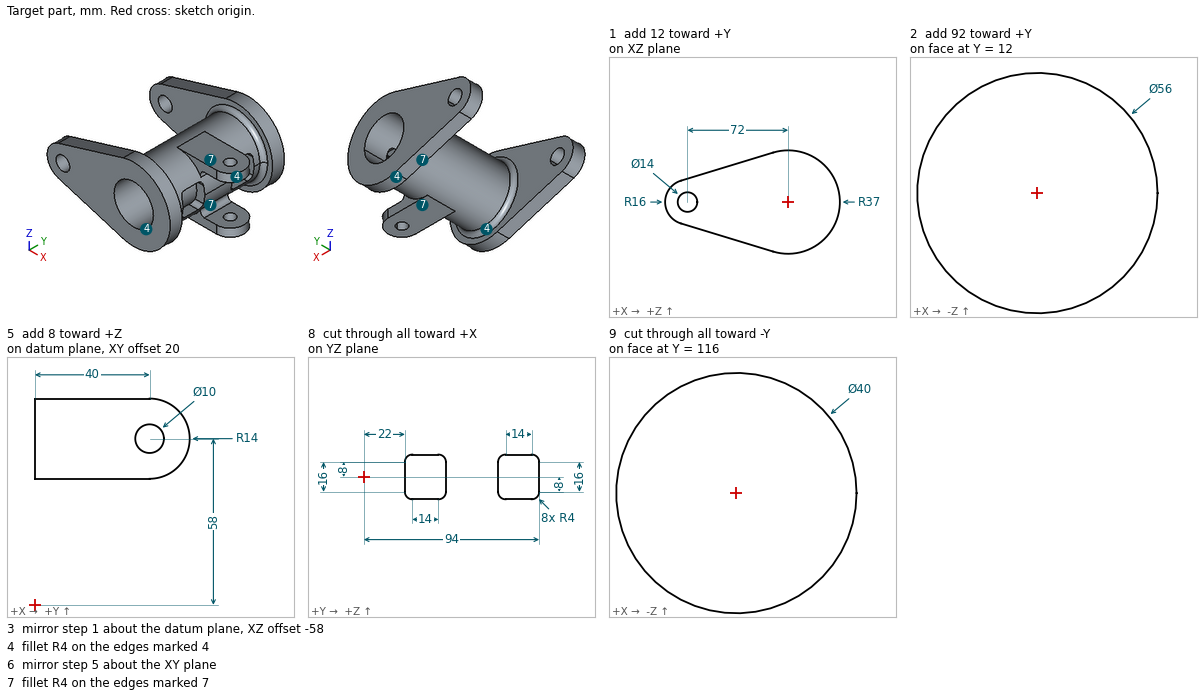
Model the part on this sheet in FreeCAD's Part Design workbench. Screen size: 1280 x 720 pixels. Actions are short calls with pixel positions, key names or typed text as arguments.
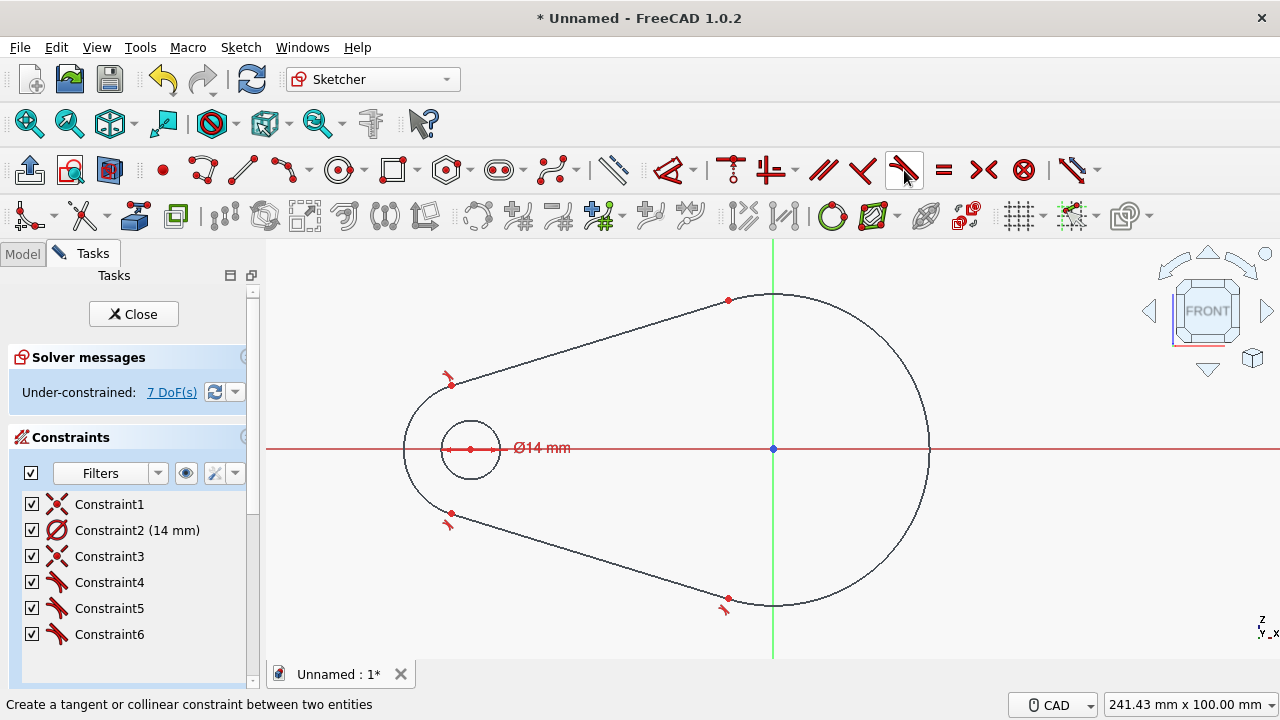
click(534, 361)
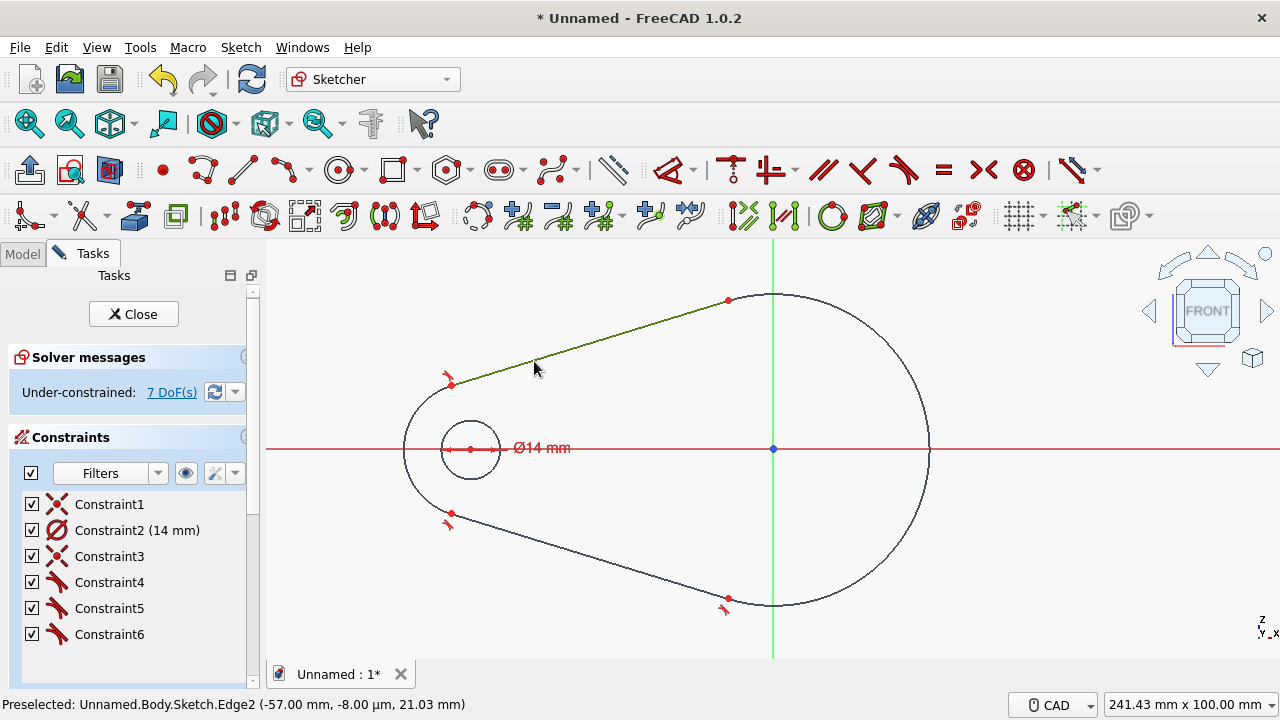
click(888, 556)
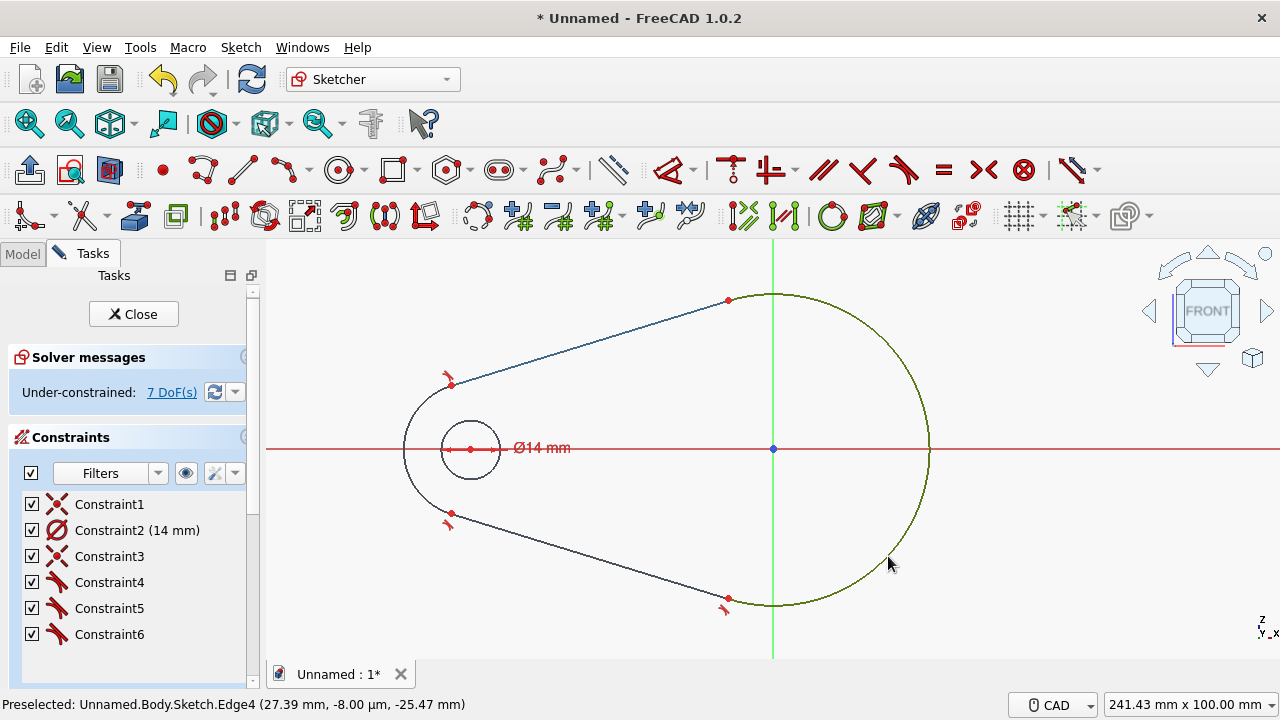
click(904, 170)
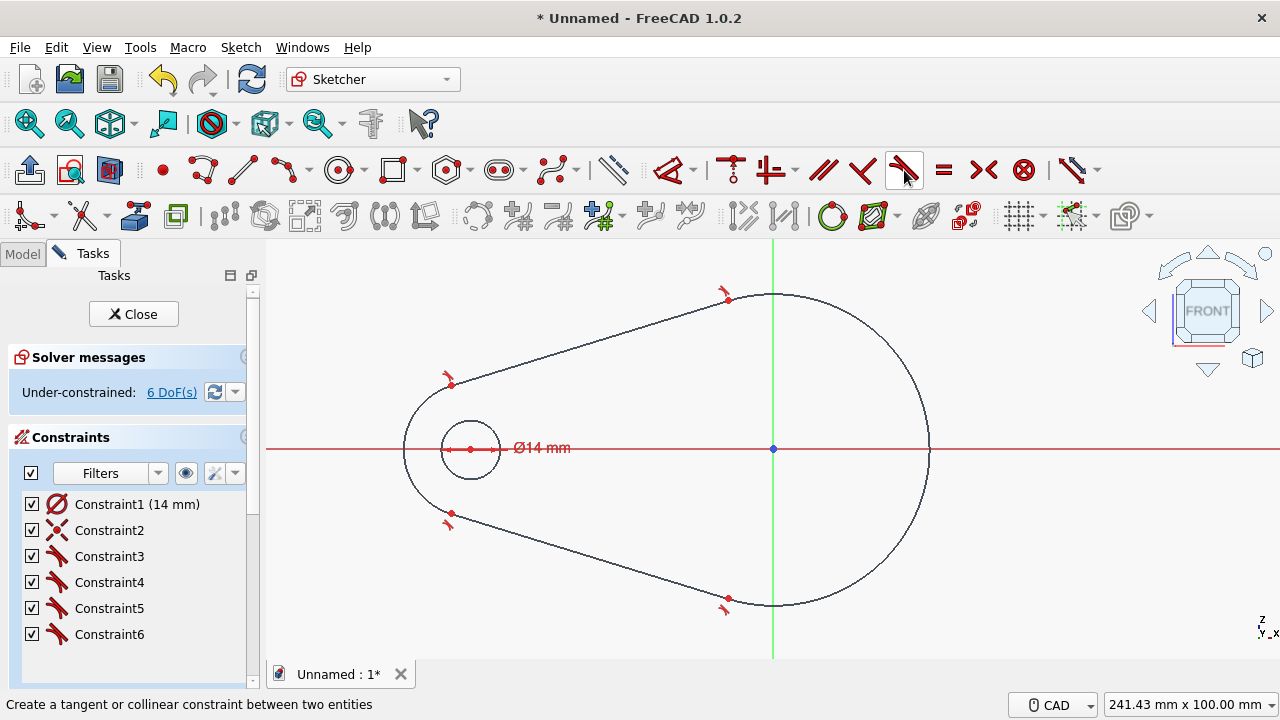
scroll(773, 449, up, 2)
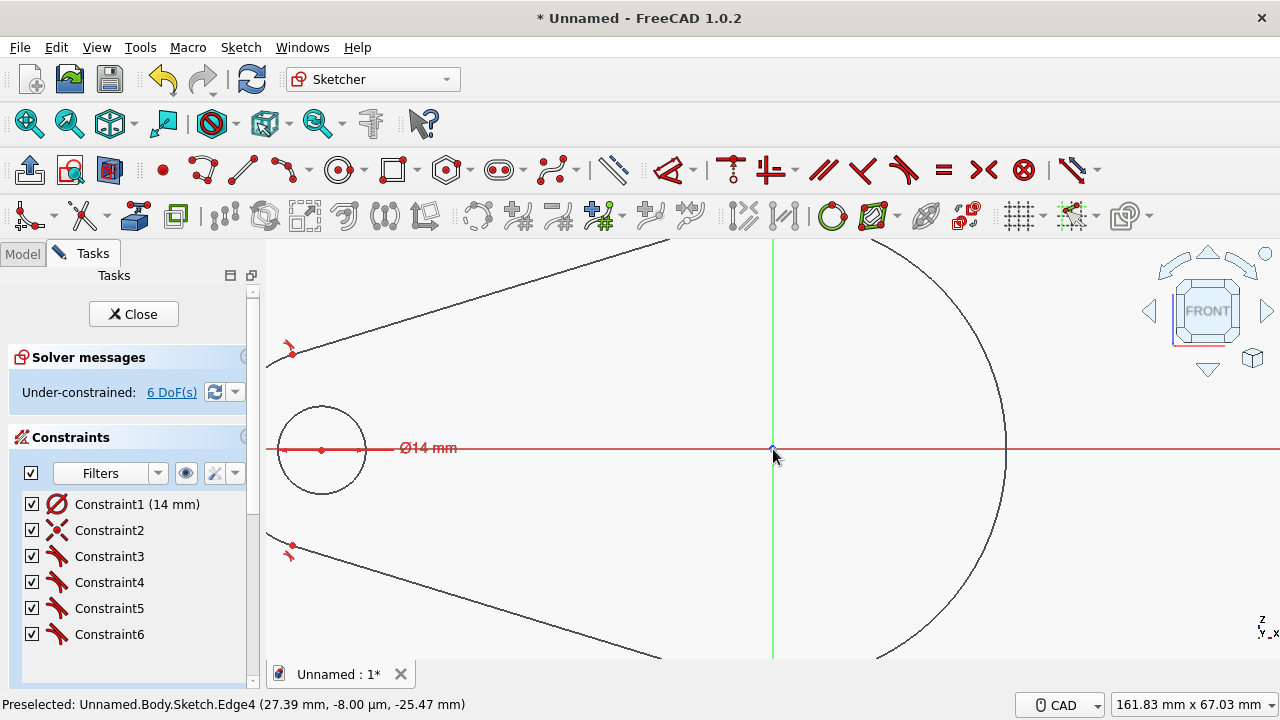
drag(763, 439, 784, 460)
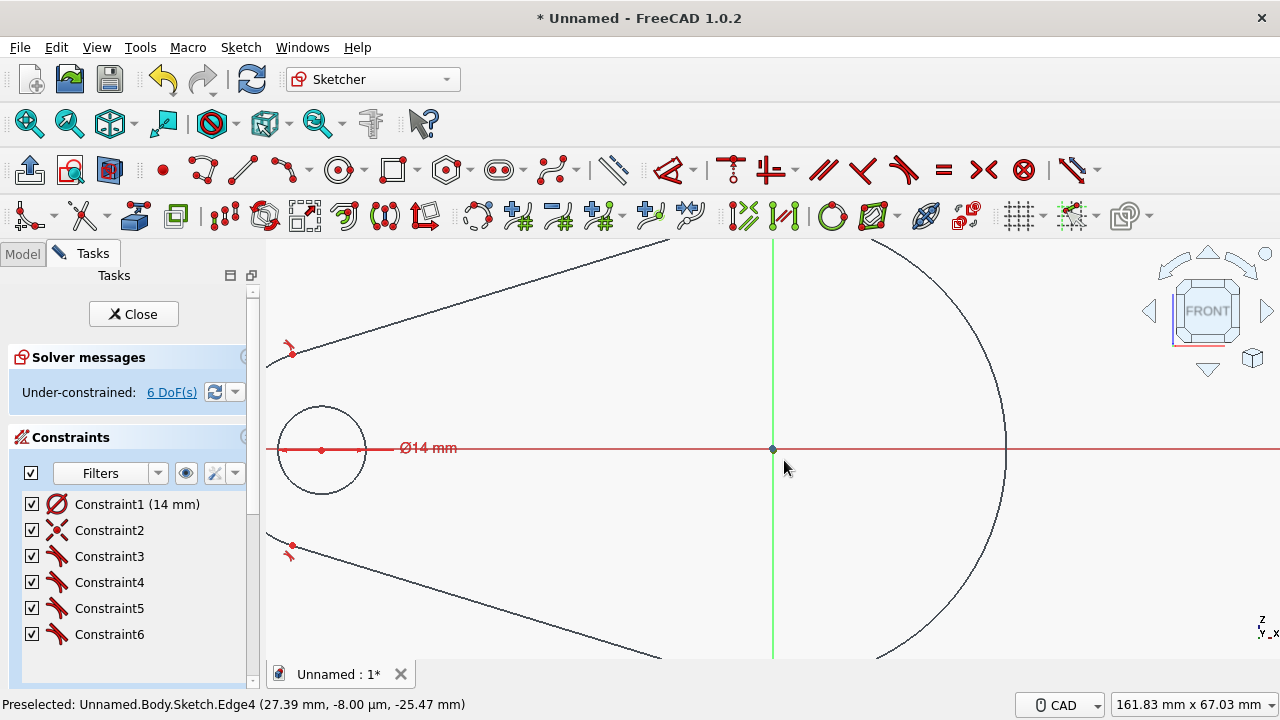
click(732, 170)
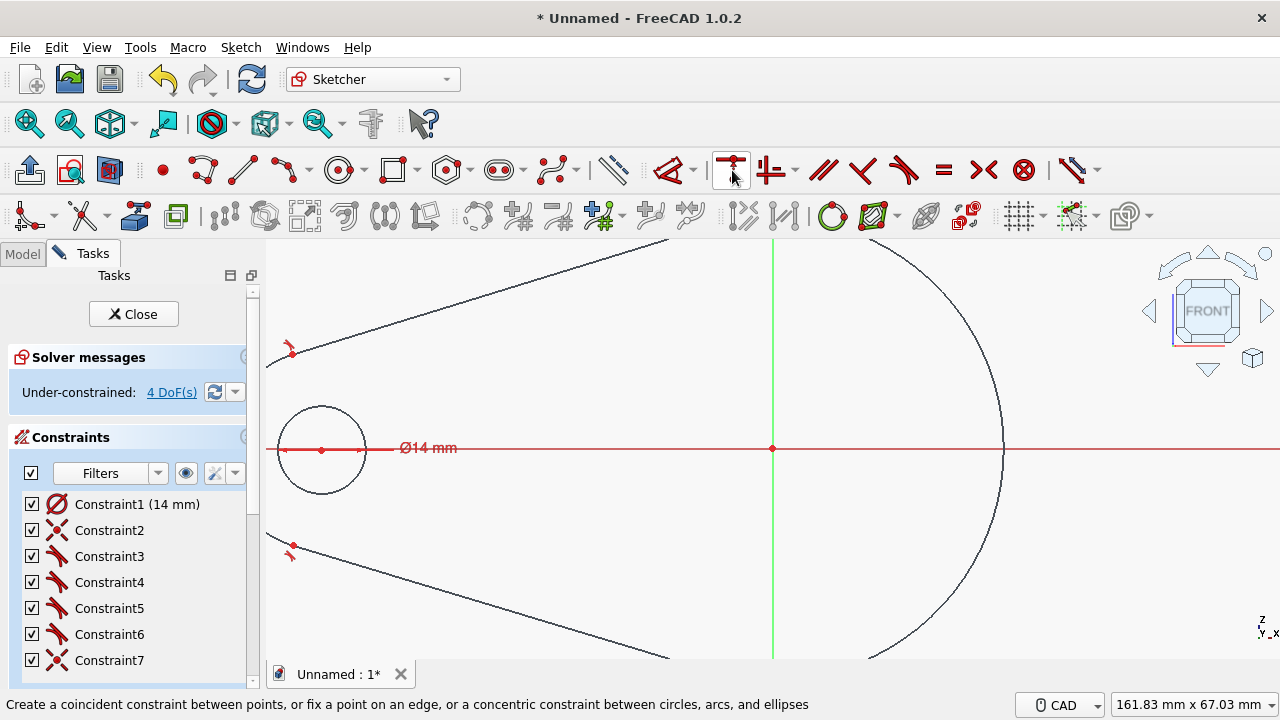
click(322, 450)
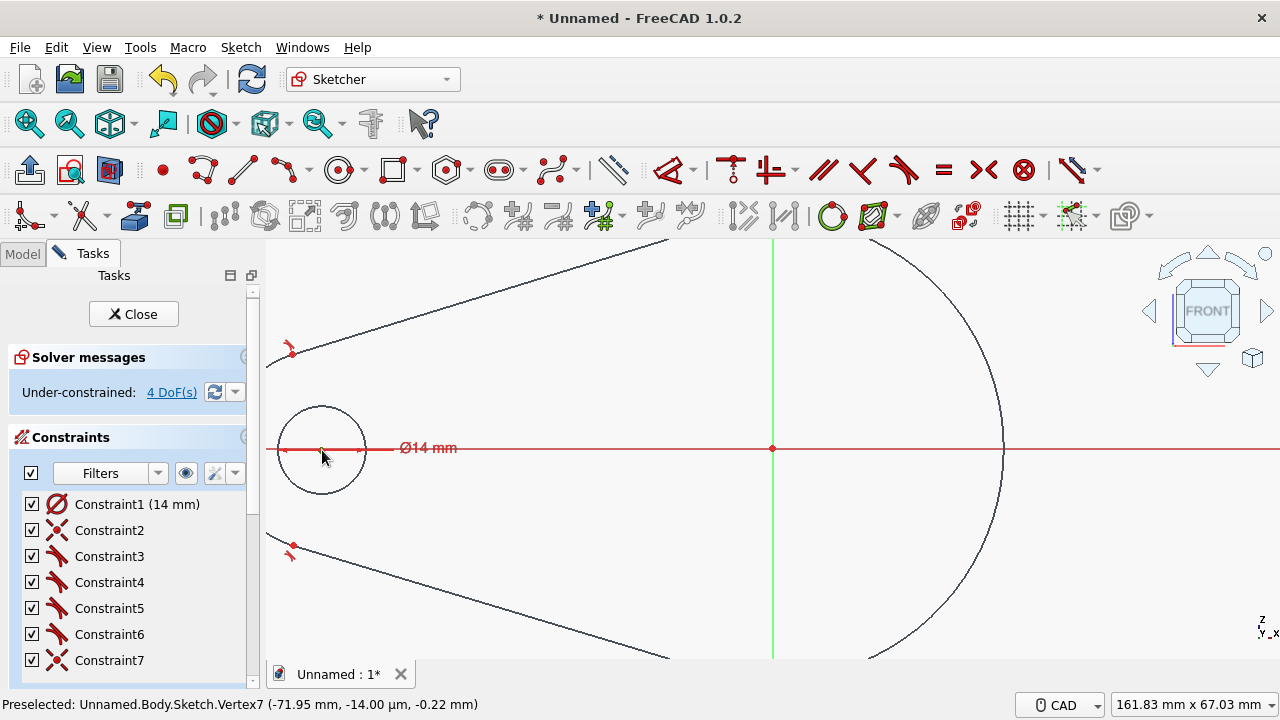
click(470, 449)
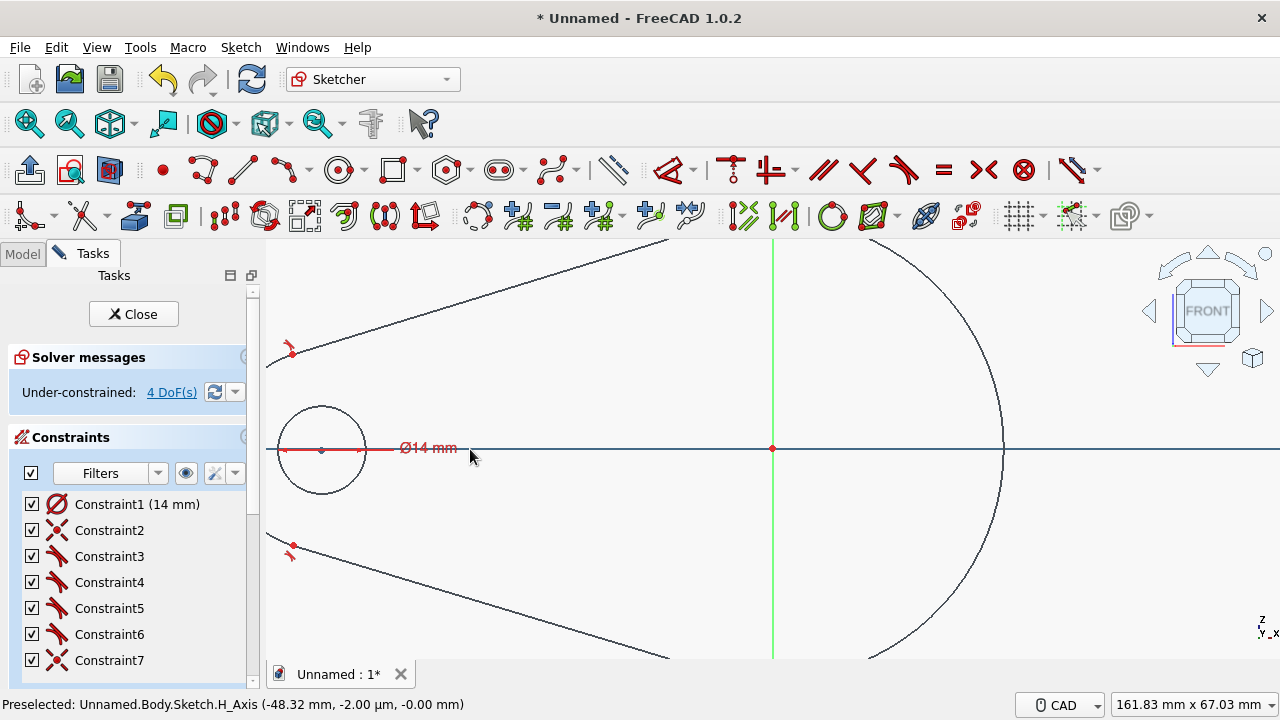
click(732, 170)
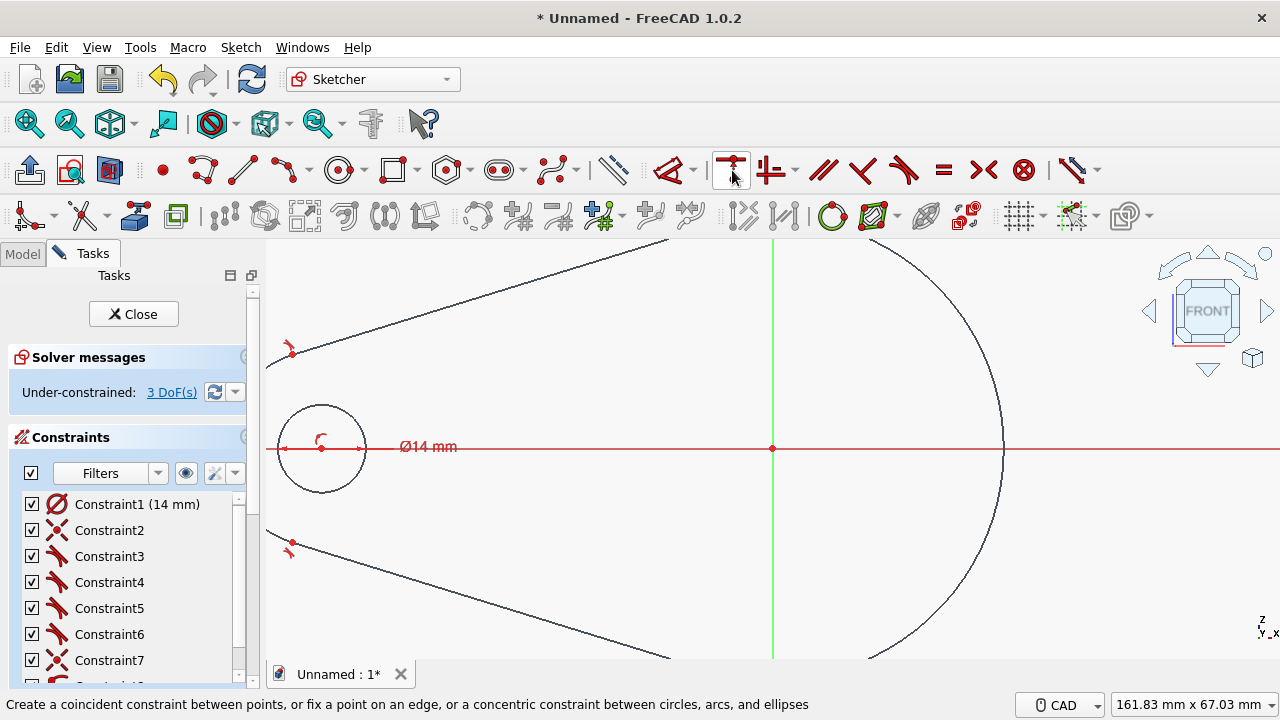
click(668, 170)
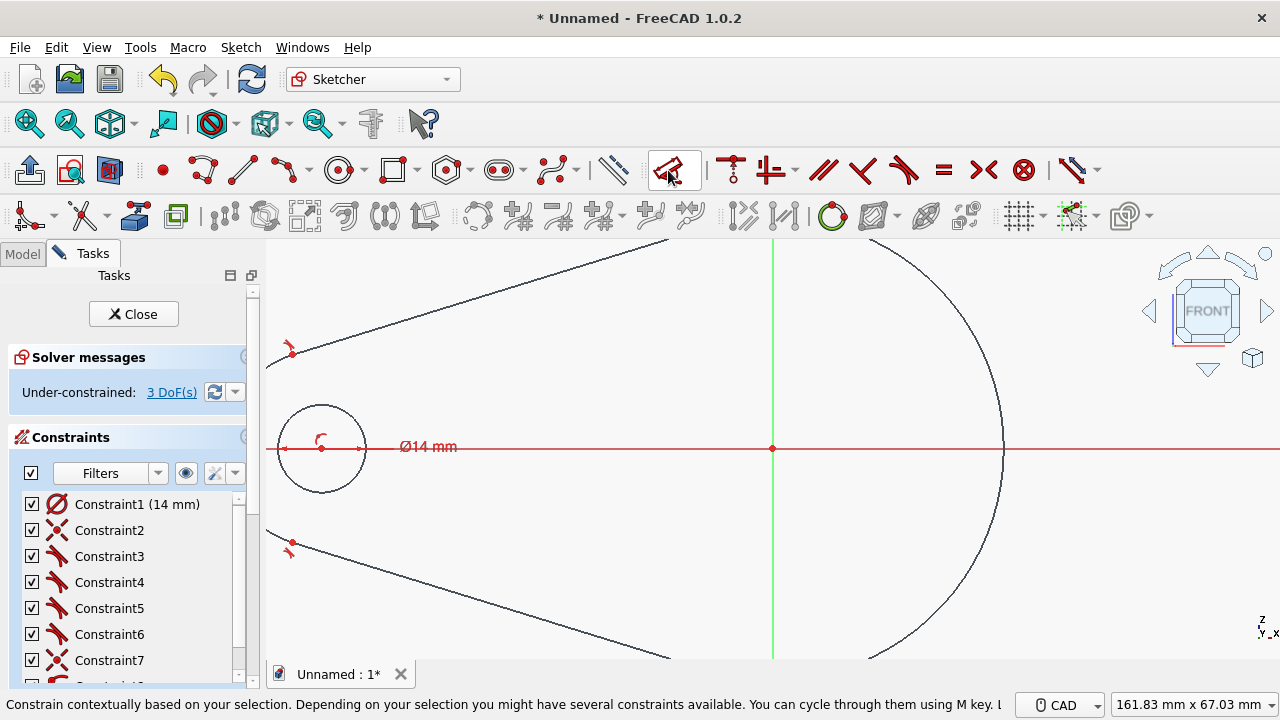
scroll(816, 449, down, 3)